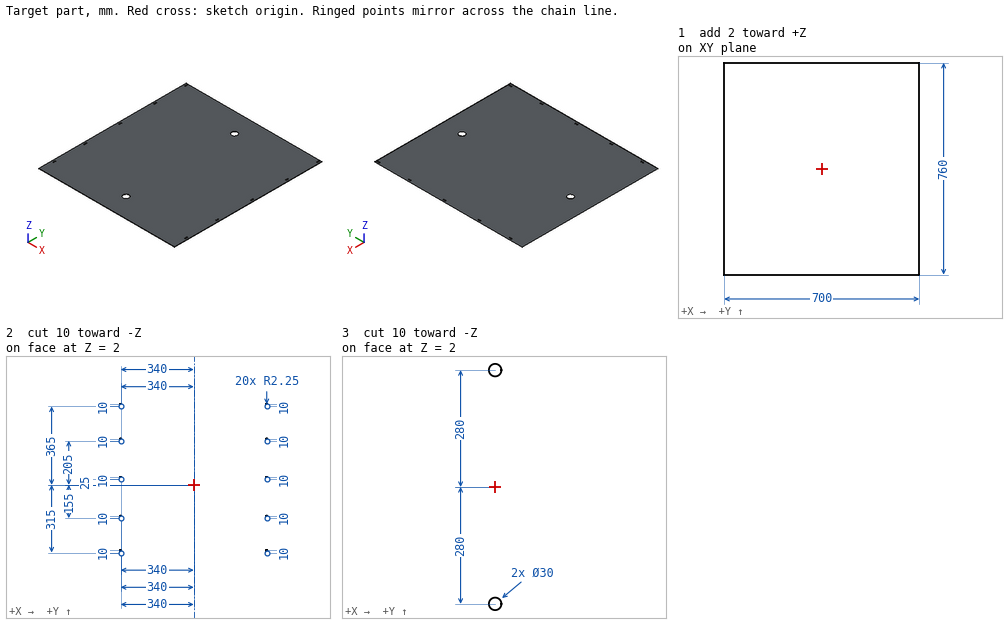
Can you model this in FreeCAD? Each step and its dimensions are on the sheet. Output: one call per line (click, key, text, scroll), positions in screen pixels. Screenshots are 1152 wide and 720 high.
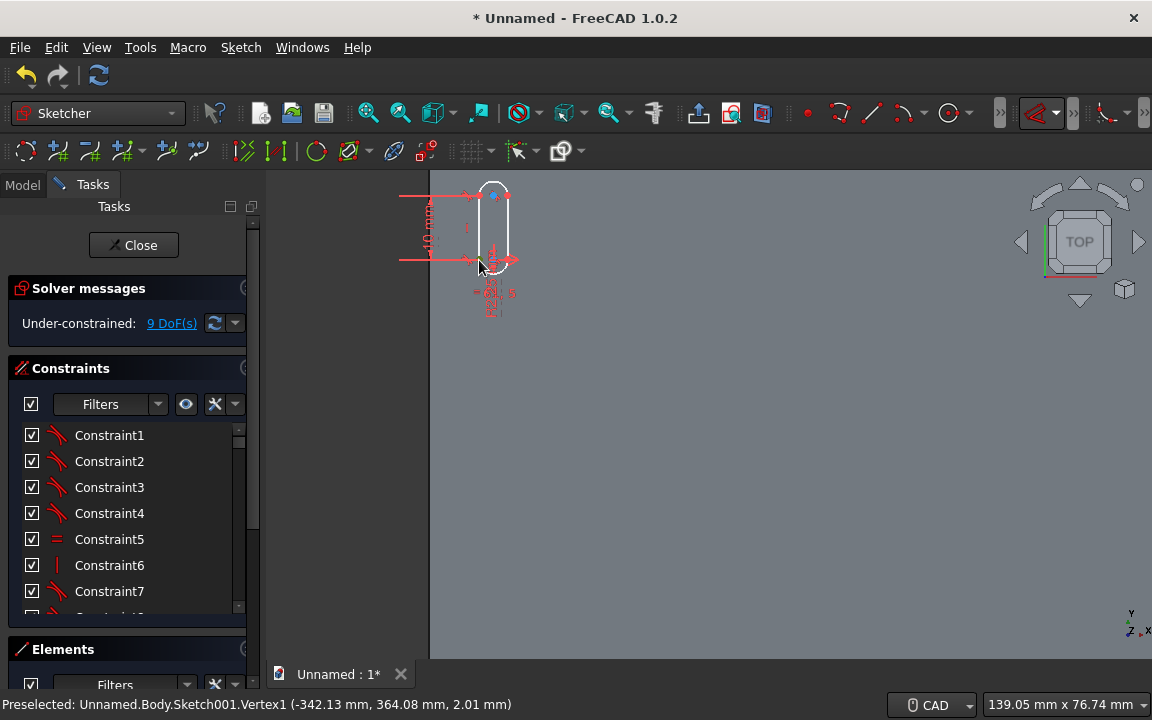
key(i)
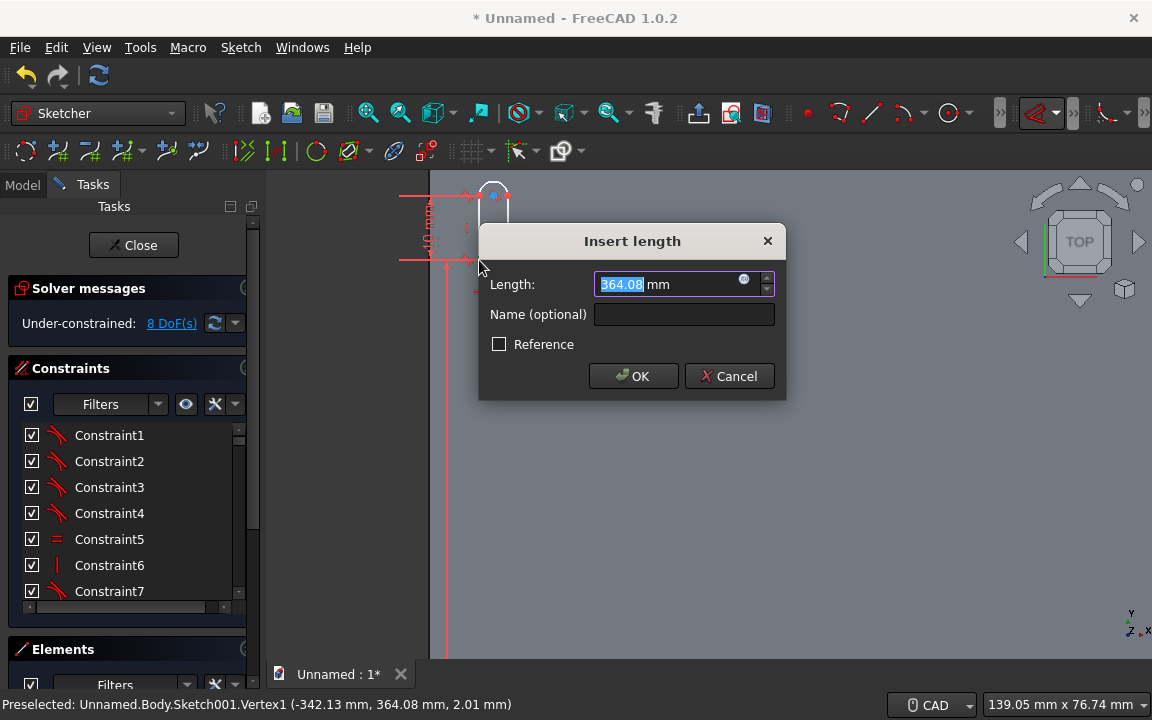
text(365)
key(Return)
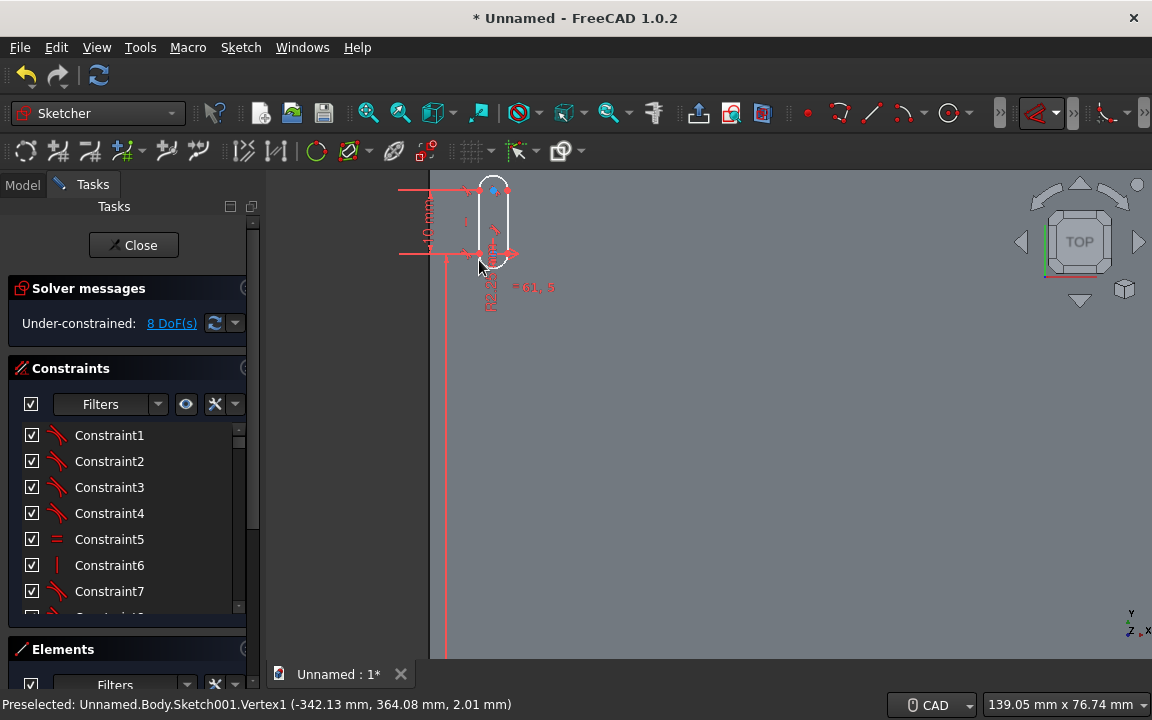
scroll(479, 256, down, 13)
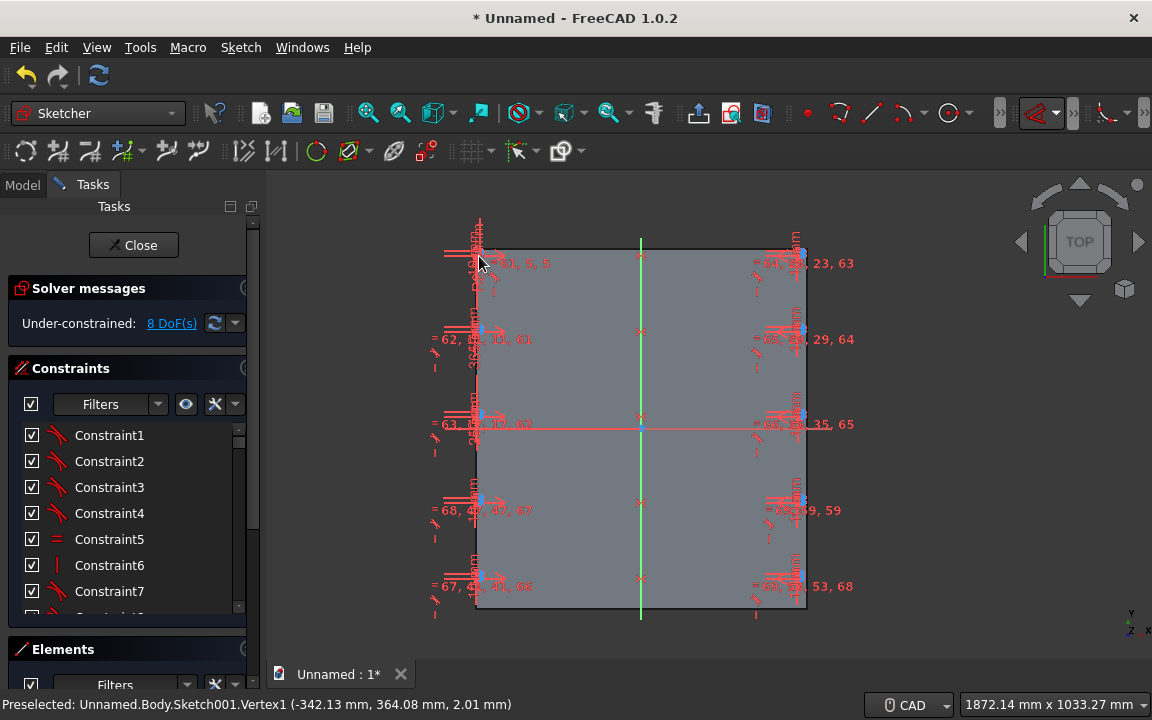
scroll(479, 332, up, 13)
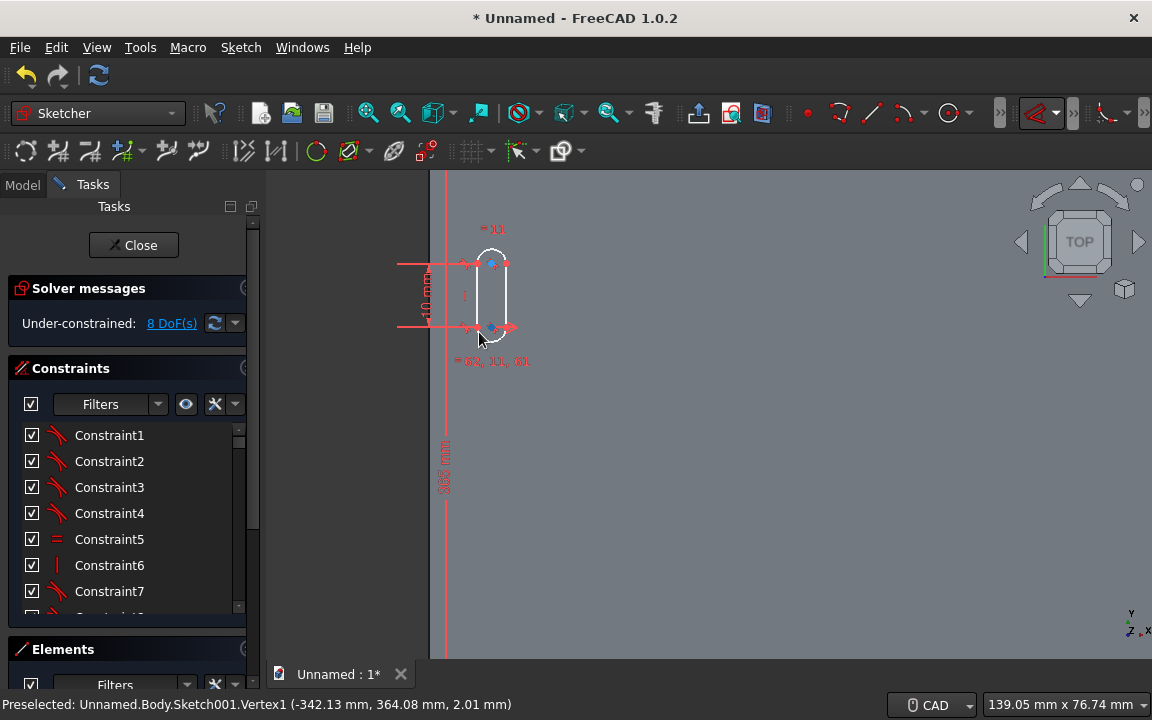
click(477, 327)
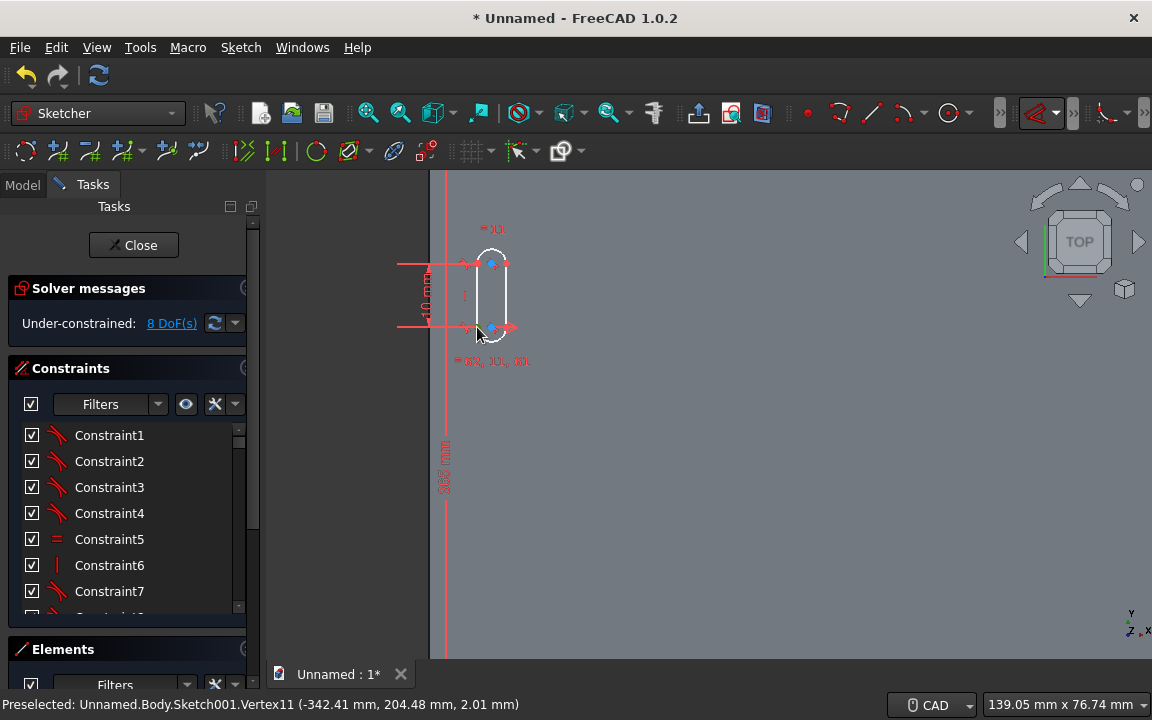
click(1058, 114)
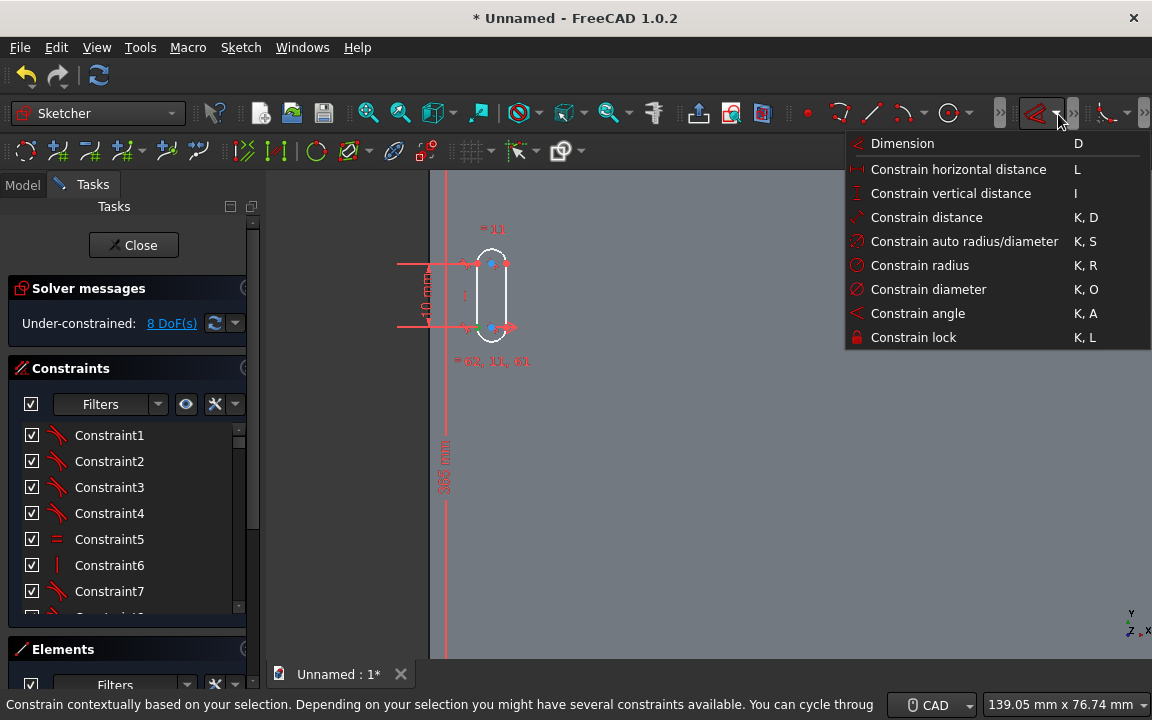
click(998, 193)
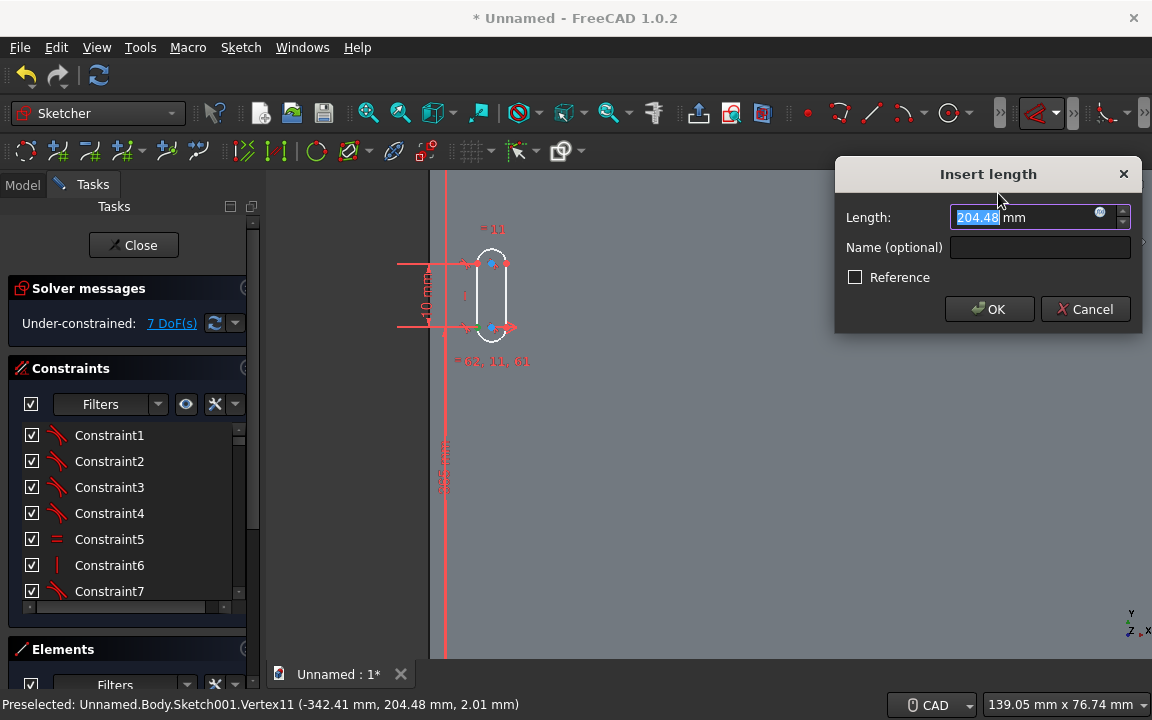
text(205)
key(Return)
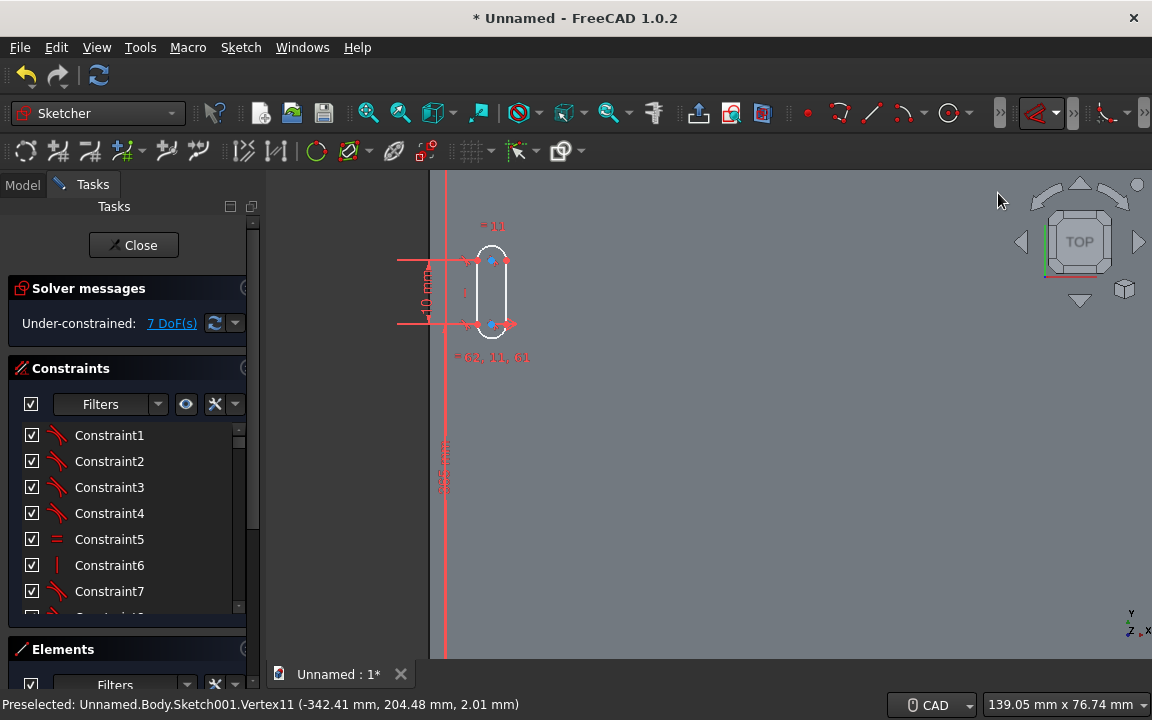
scroll(479, 332, down, 13)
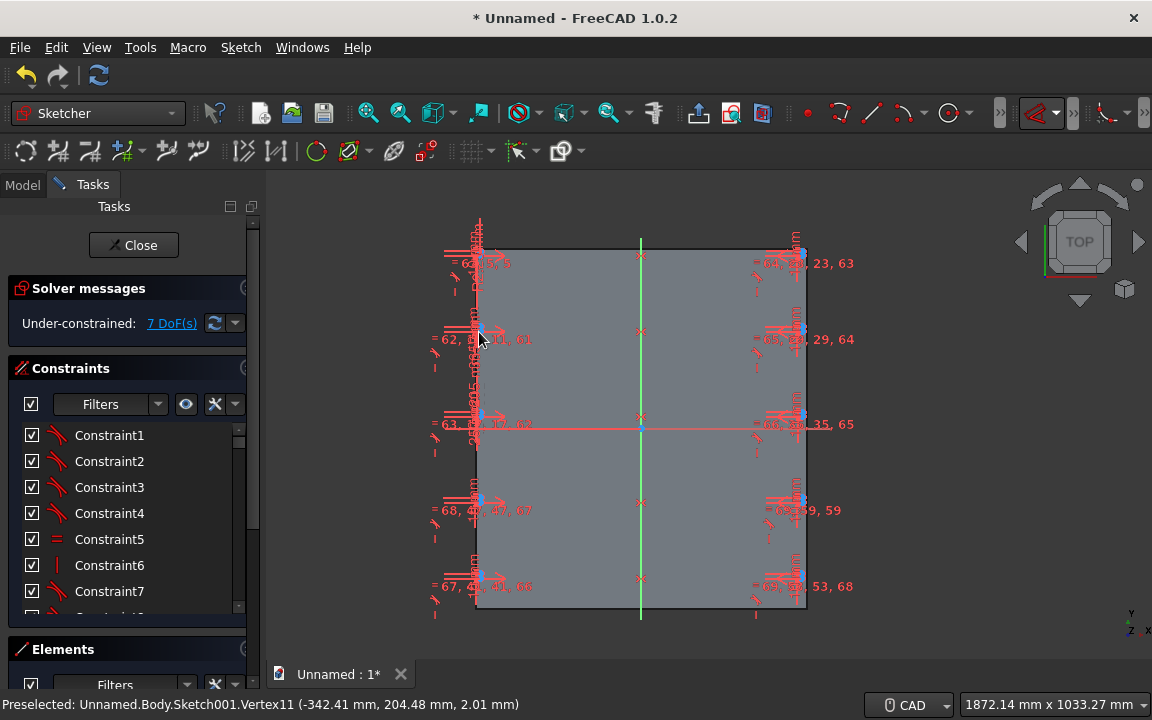
scroll(480, 579, up, 13)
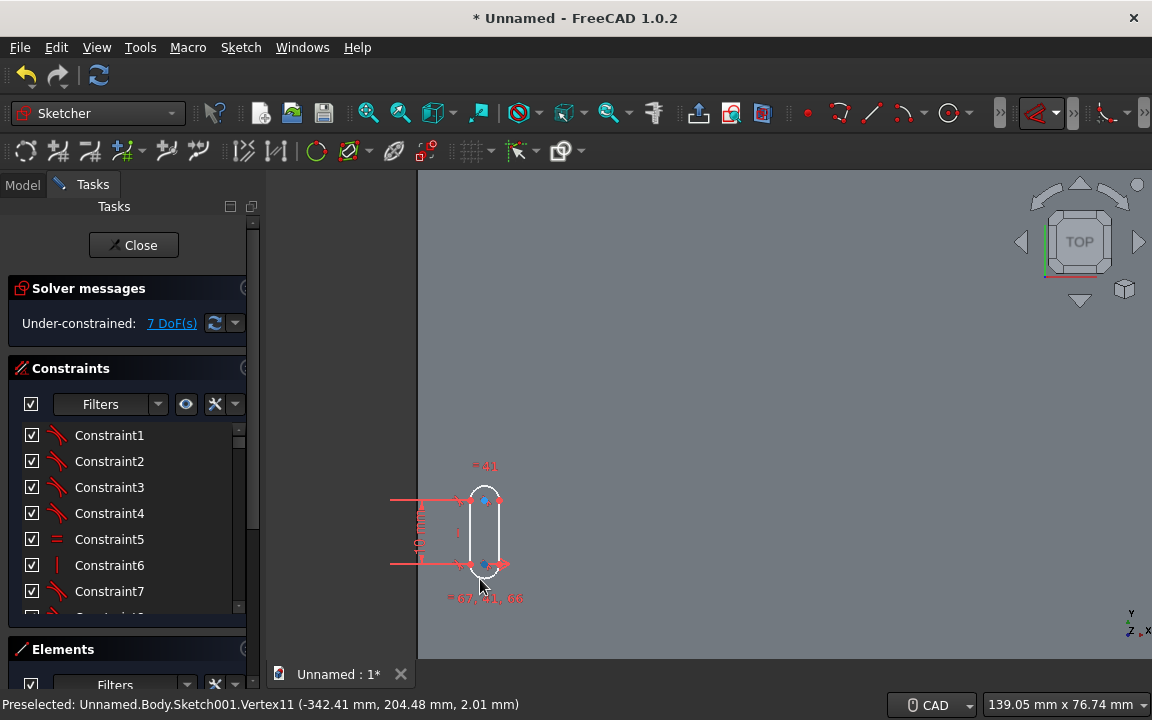
click(470, 564)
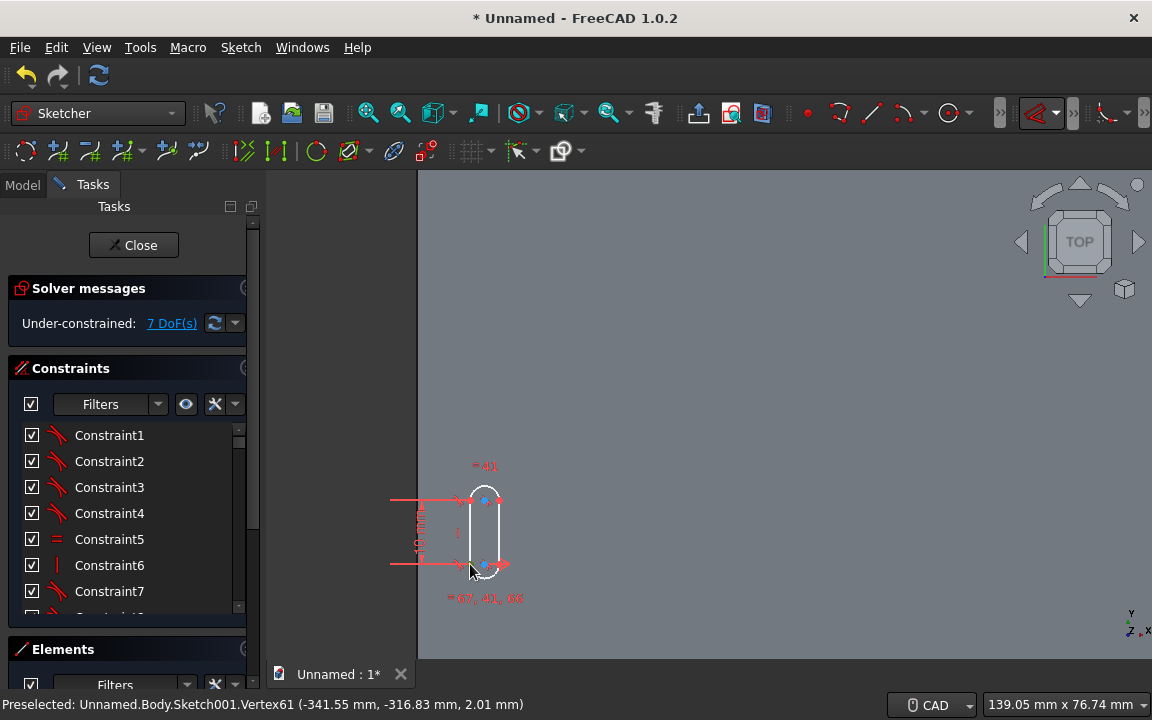
click(1058, 114)